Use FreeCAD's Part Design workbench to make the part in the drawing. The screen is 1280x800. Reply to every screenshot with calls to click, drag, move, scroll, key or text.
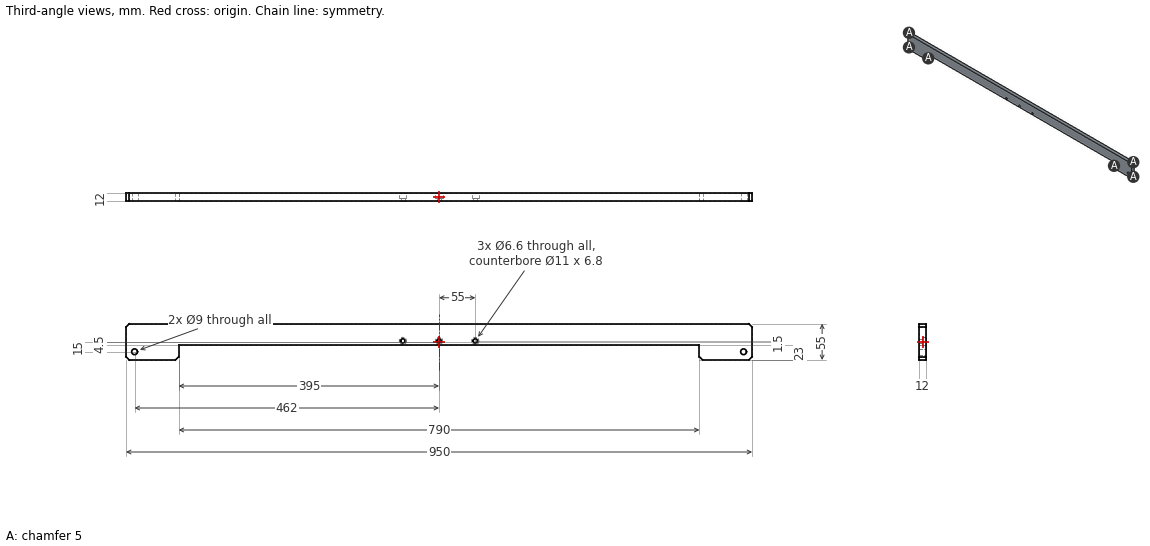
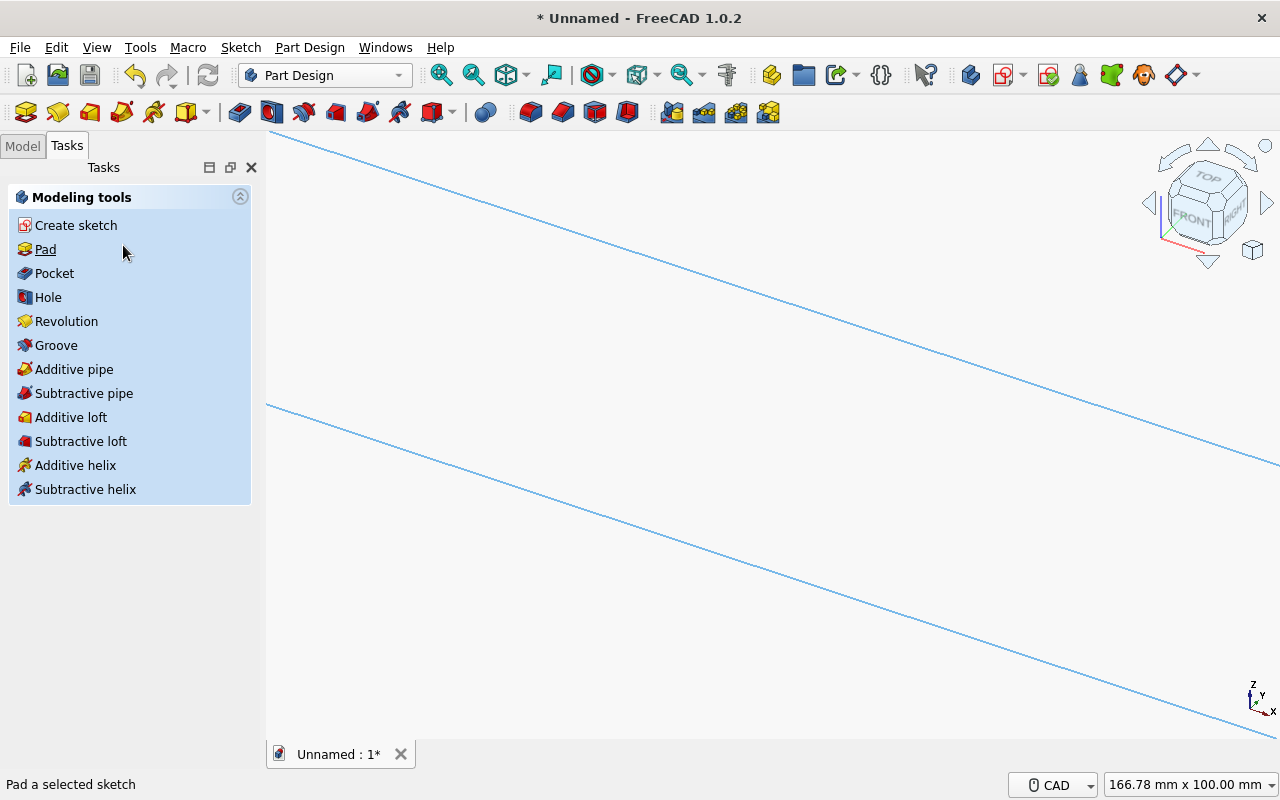
click(26, 112)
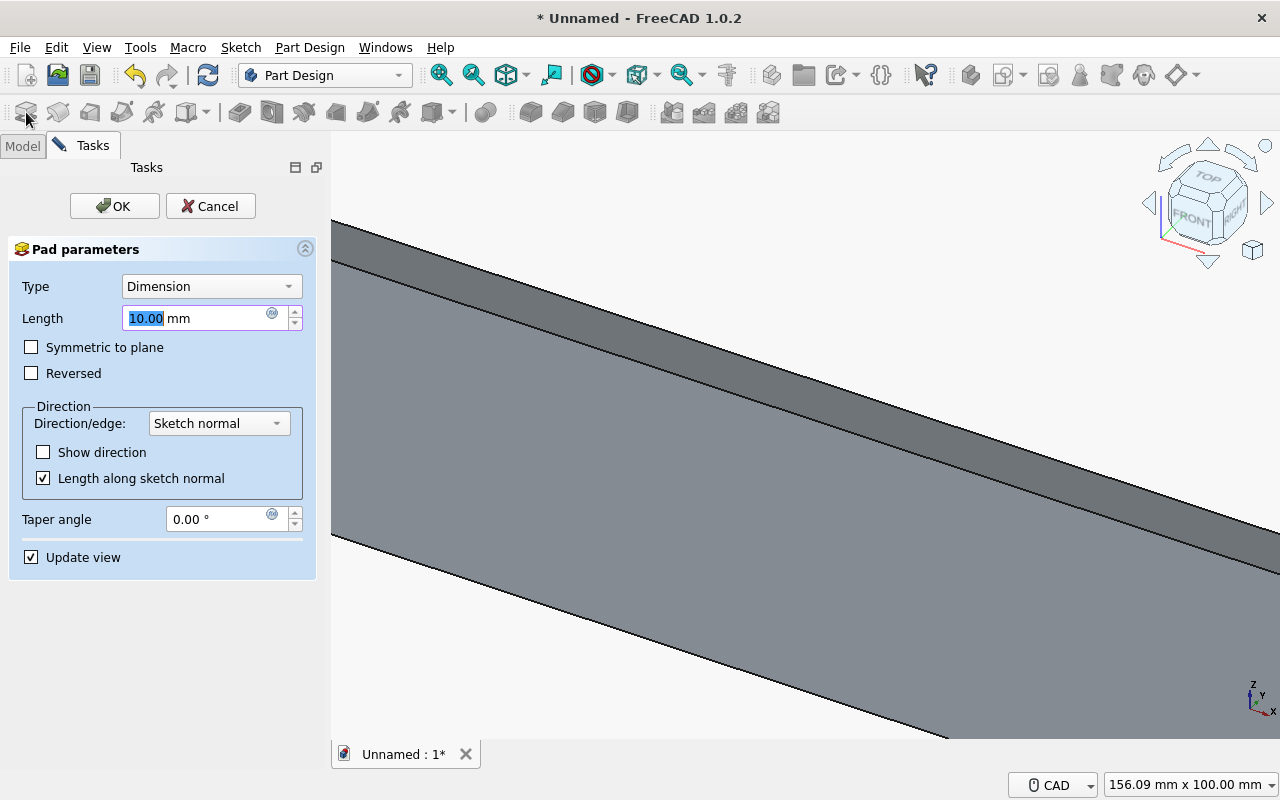
text(12)
key(Tab)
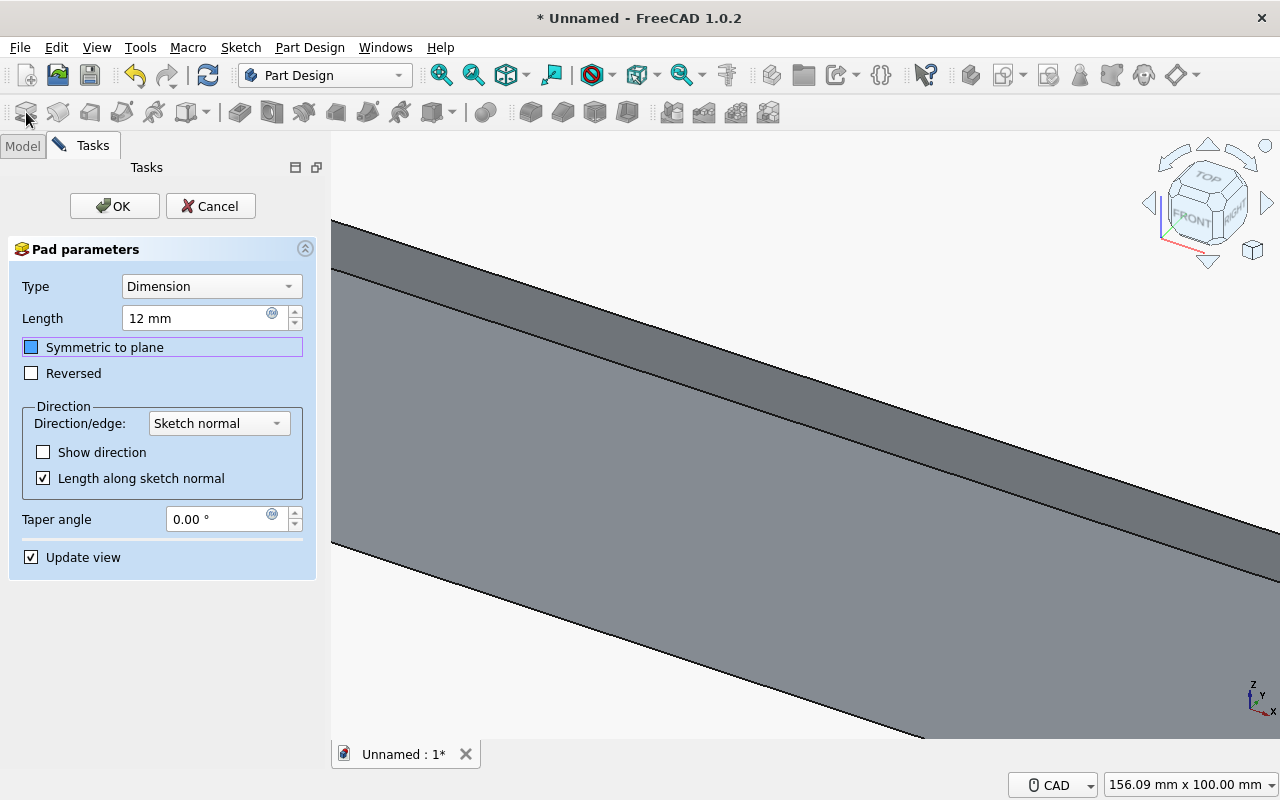
click(30, 347)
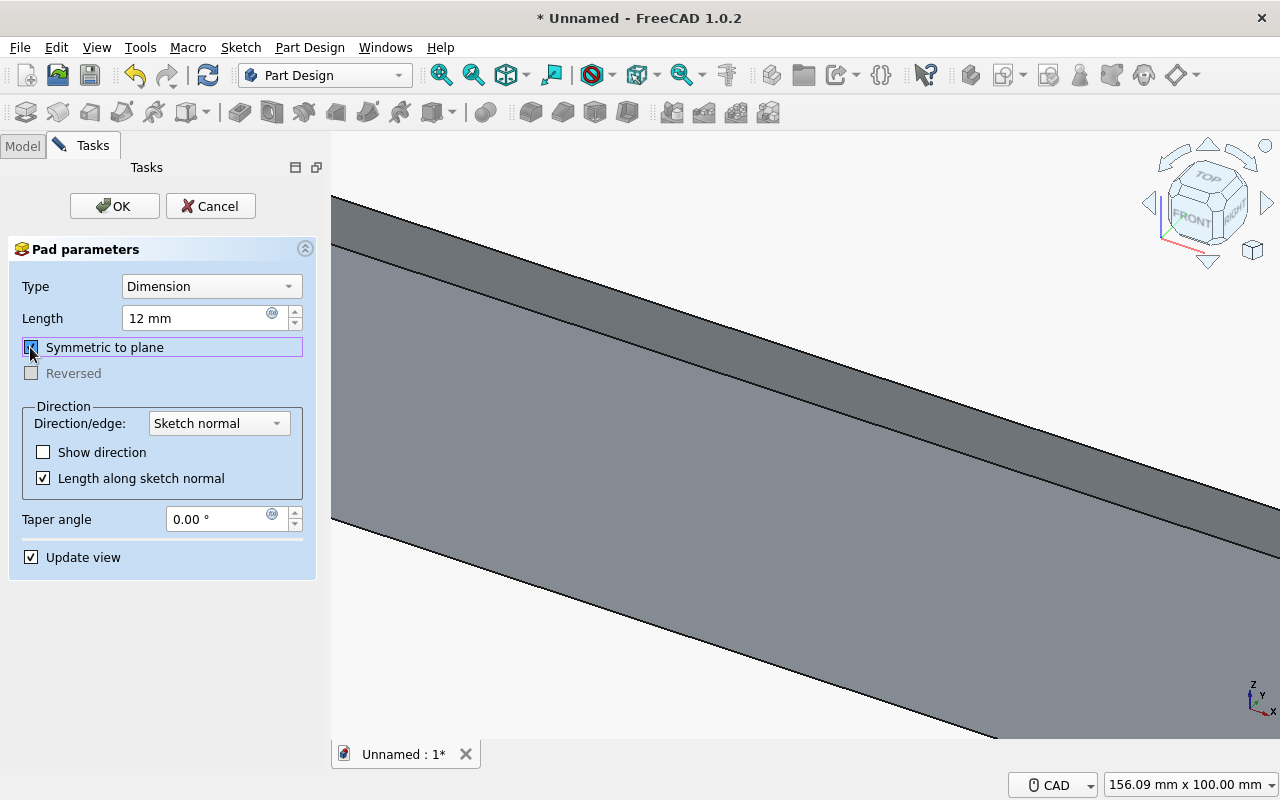
click(115, 206)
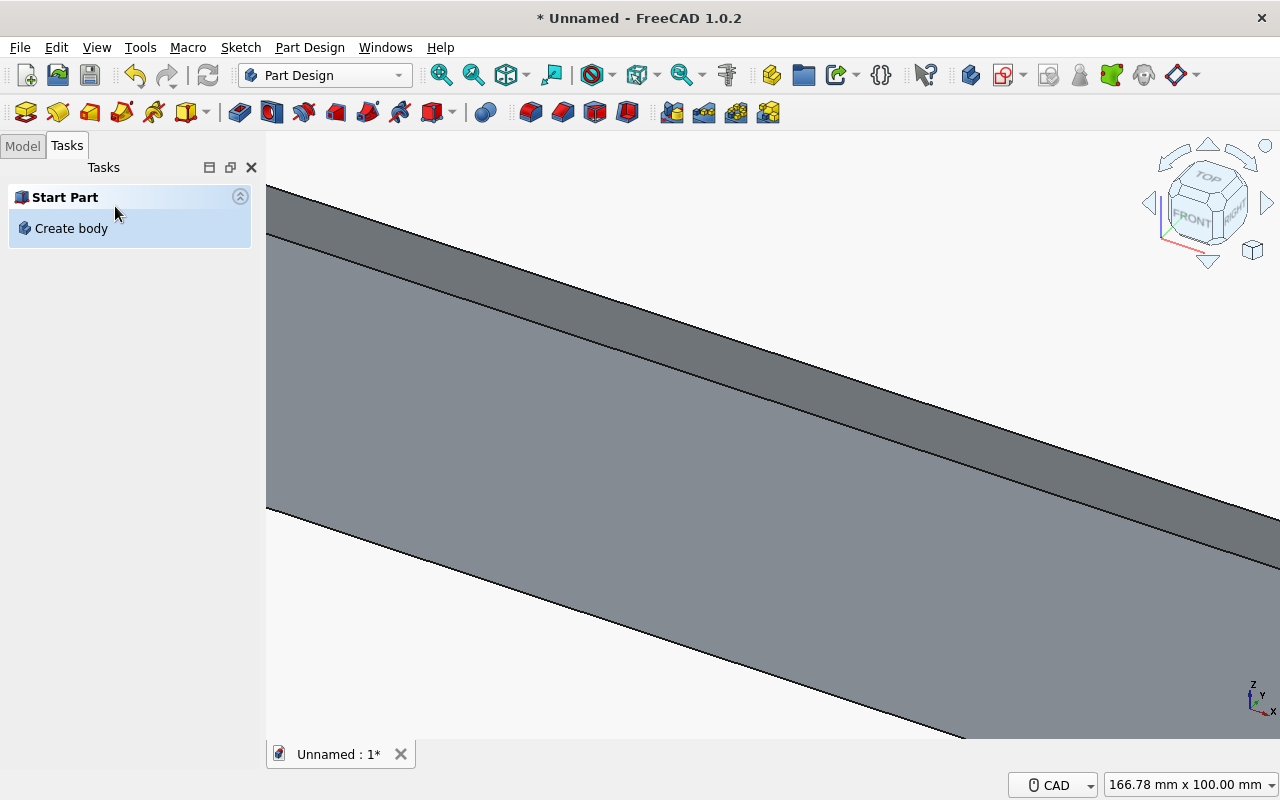
key(v)
key(f)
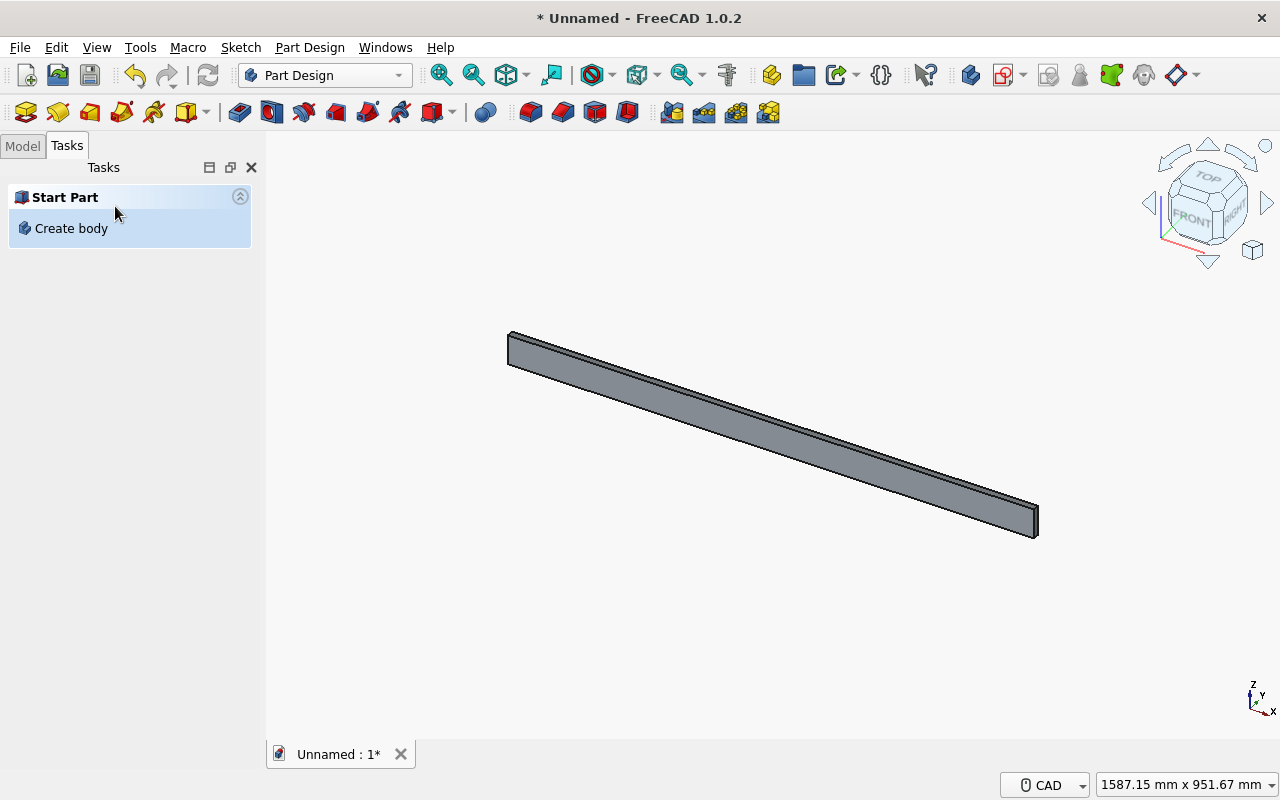
key(4)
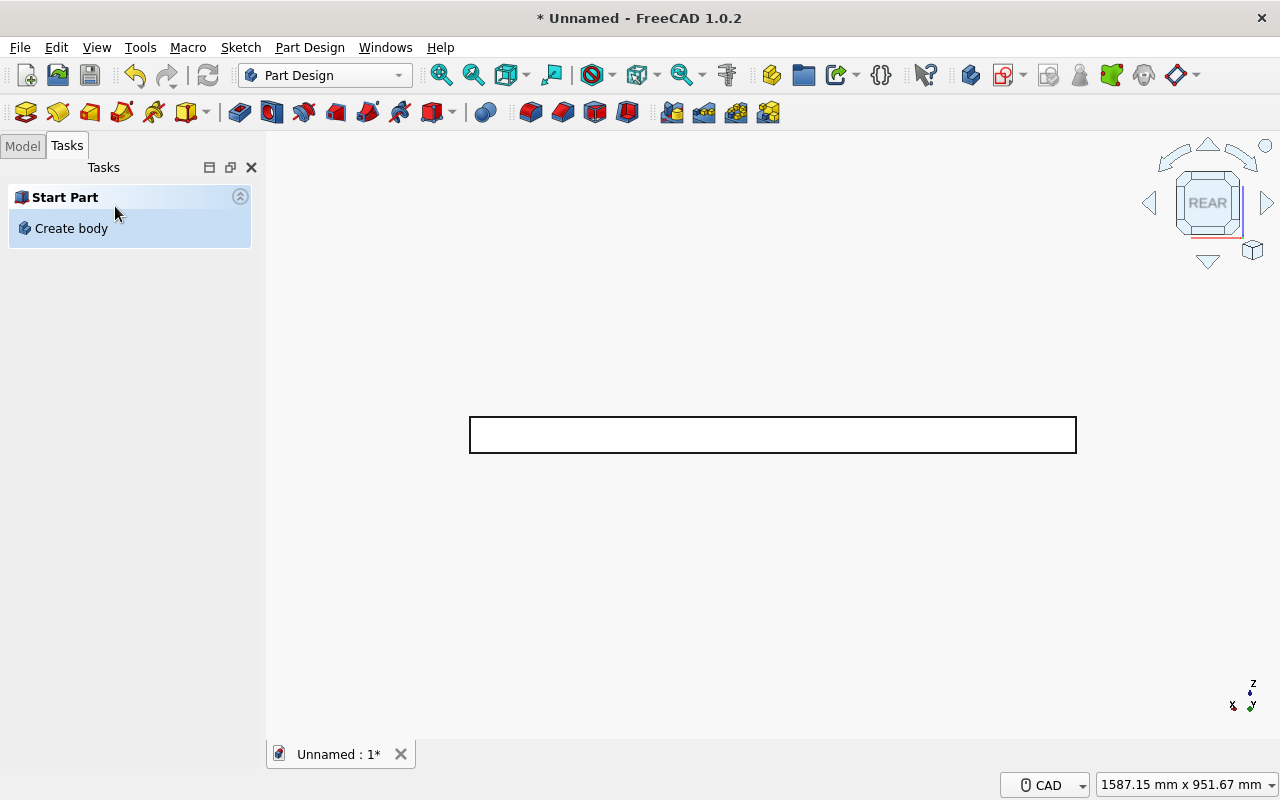
click(513, 434)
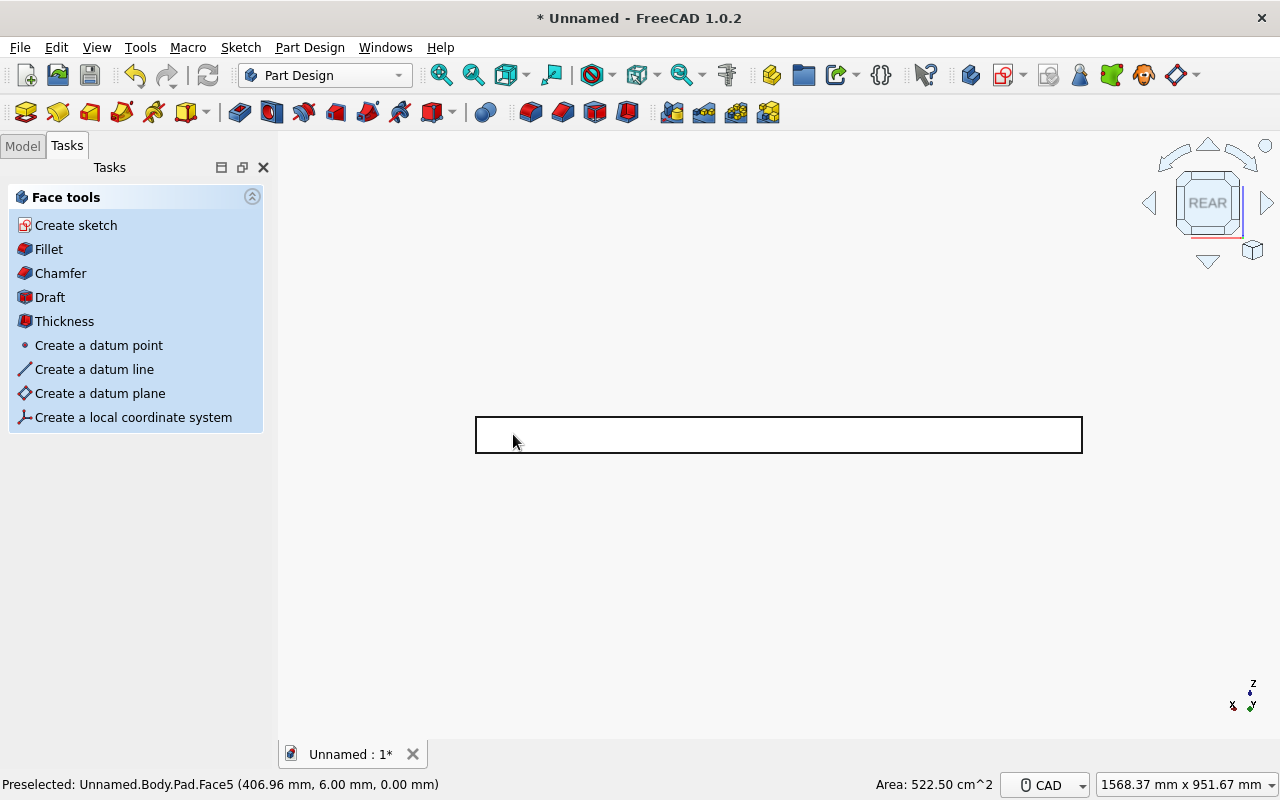
click(1004, 76)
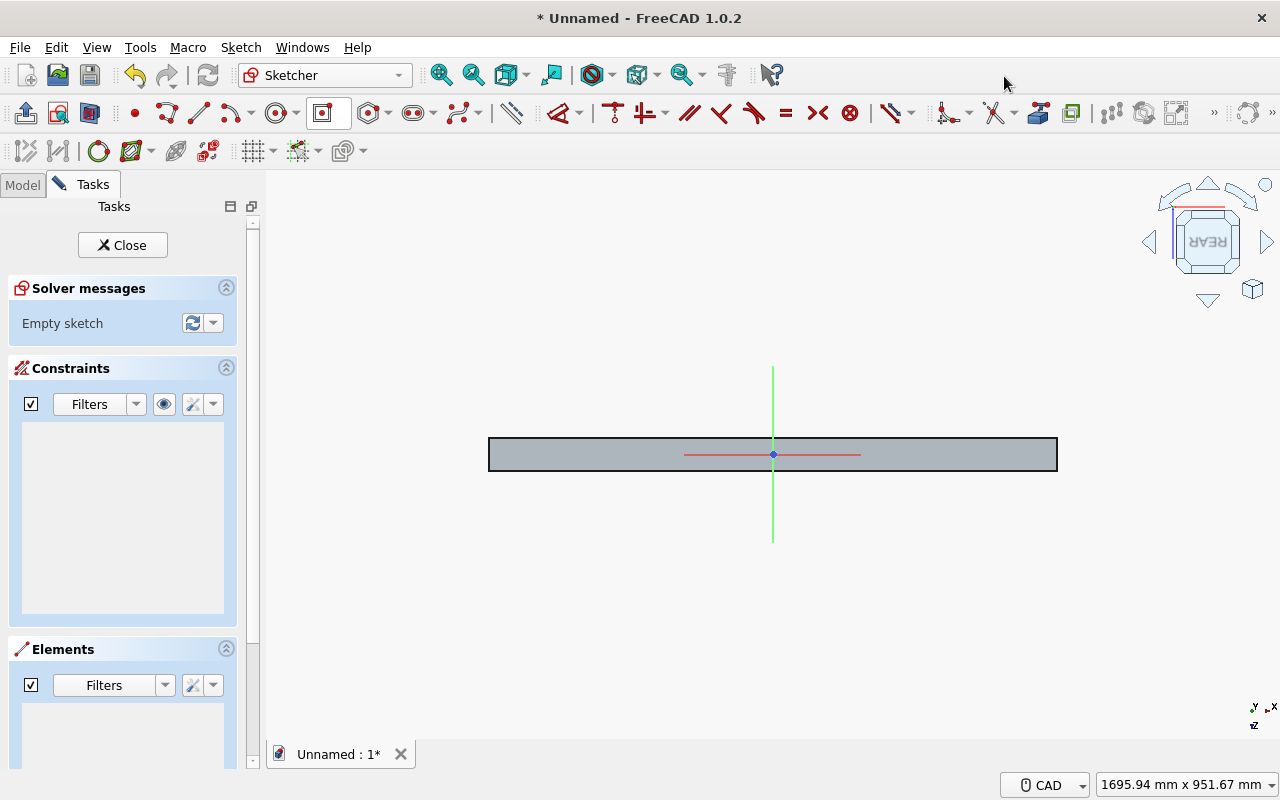
key(g)
key(r)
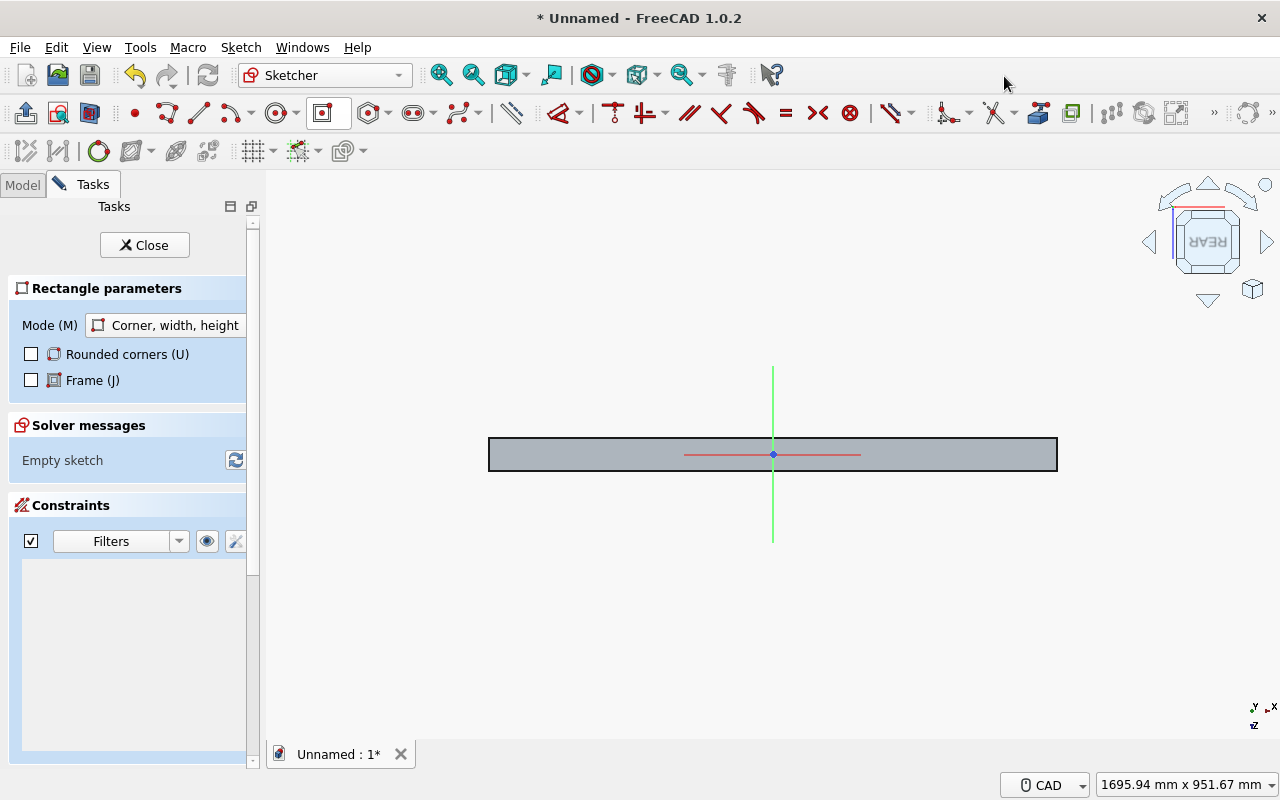
click(537, 438)